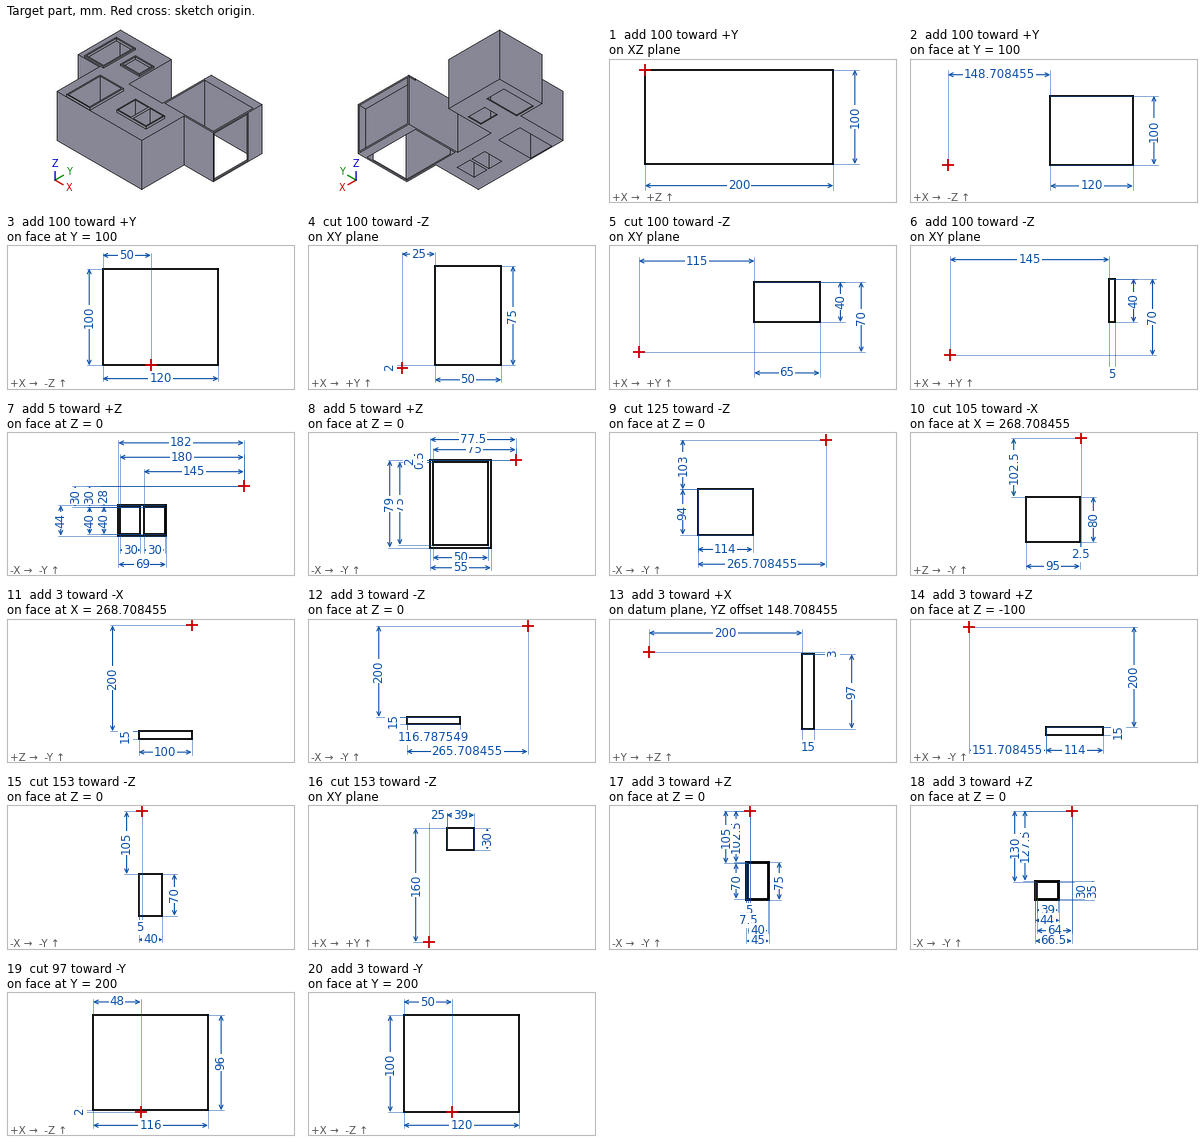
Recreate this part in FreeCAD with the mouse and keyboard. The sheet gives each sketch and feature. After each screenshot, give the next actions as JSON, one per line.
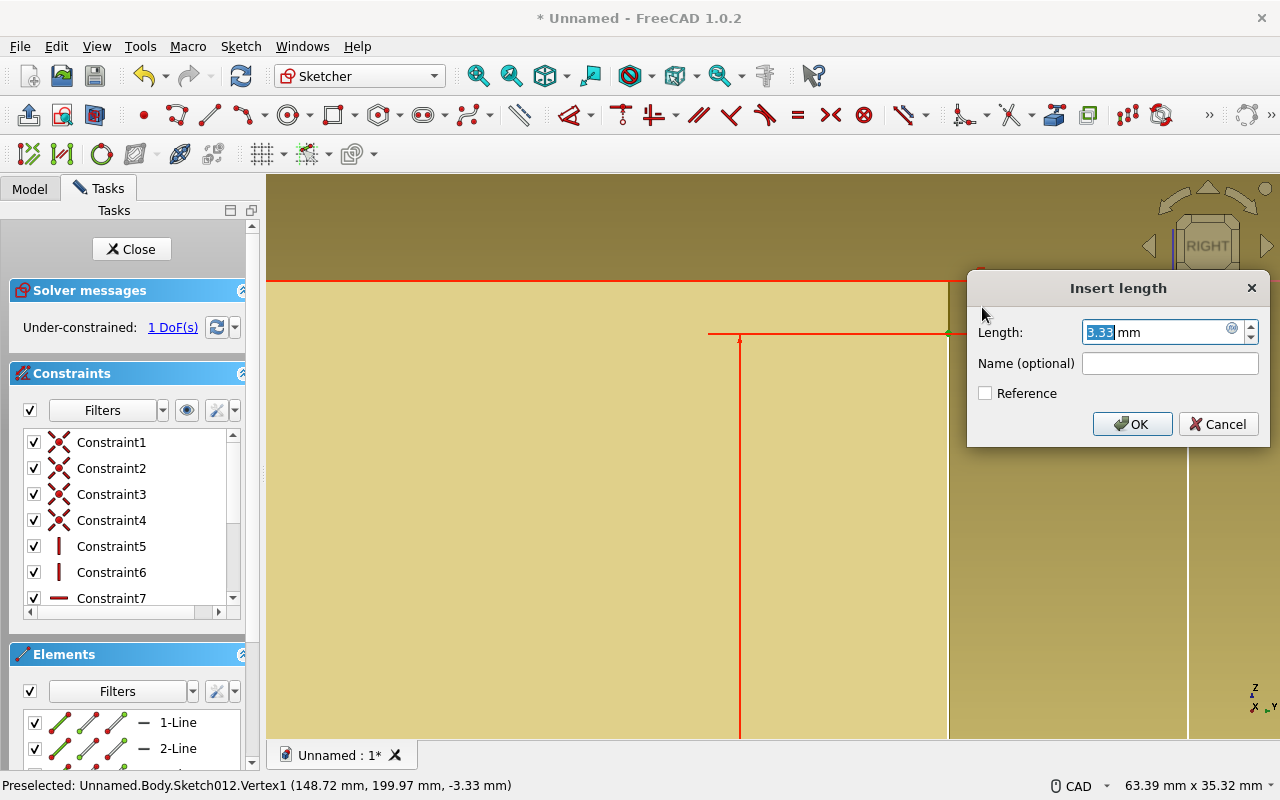
{"action": "type", "text": "3"}
{"action": "key", "text": "Return"}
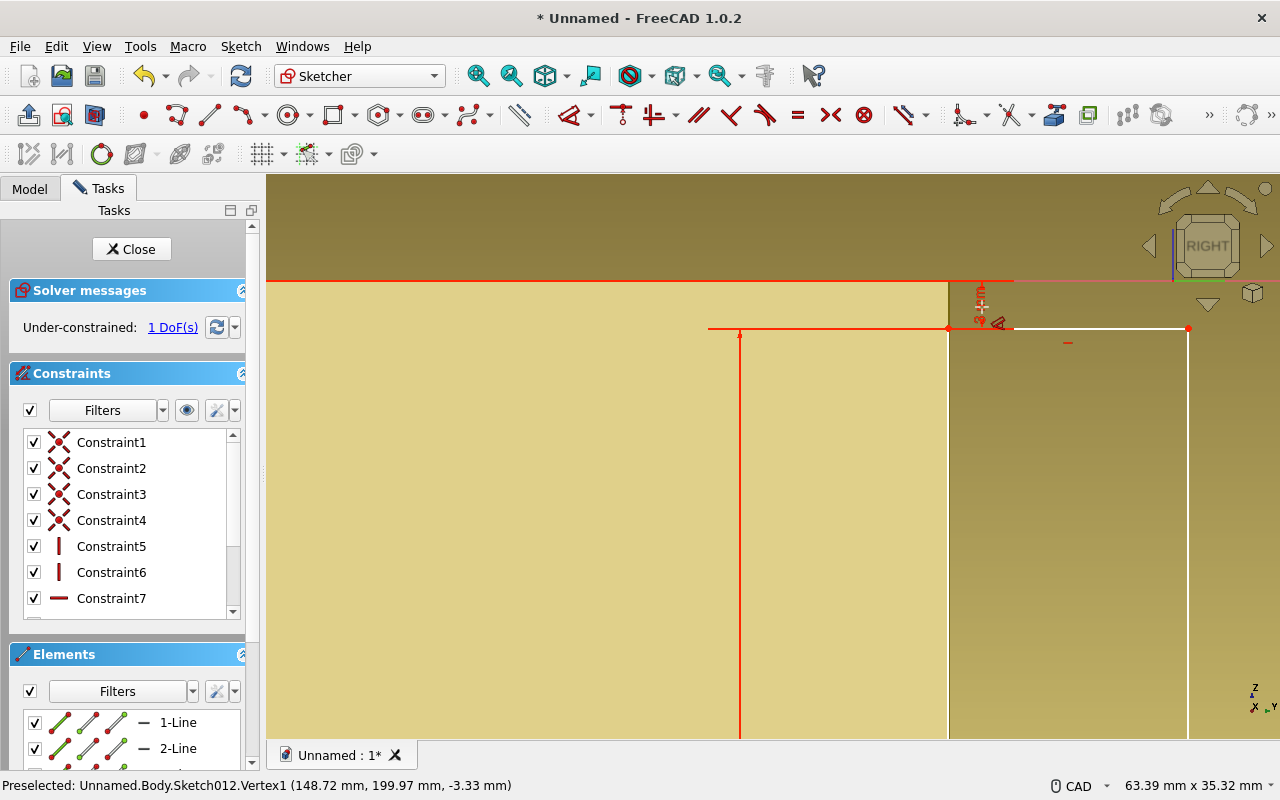
{"action": "scroll", "coordinate": [949, 333], "scroll_direction": "down", "scroll_amount": 9}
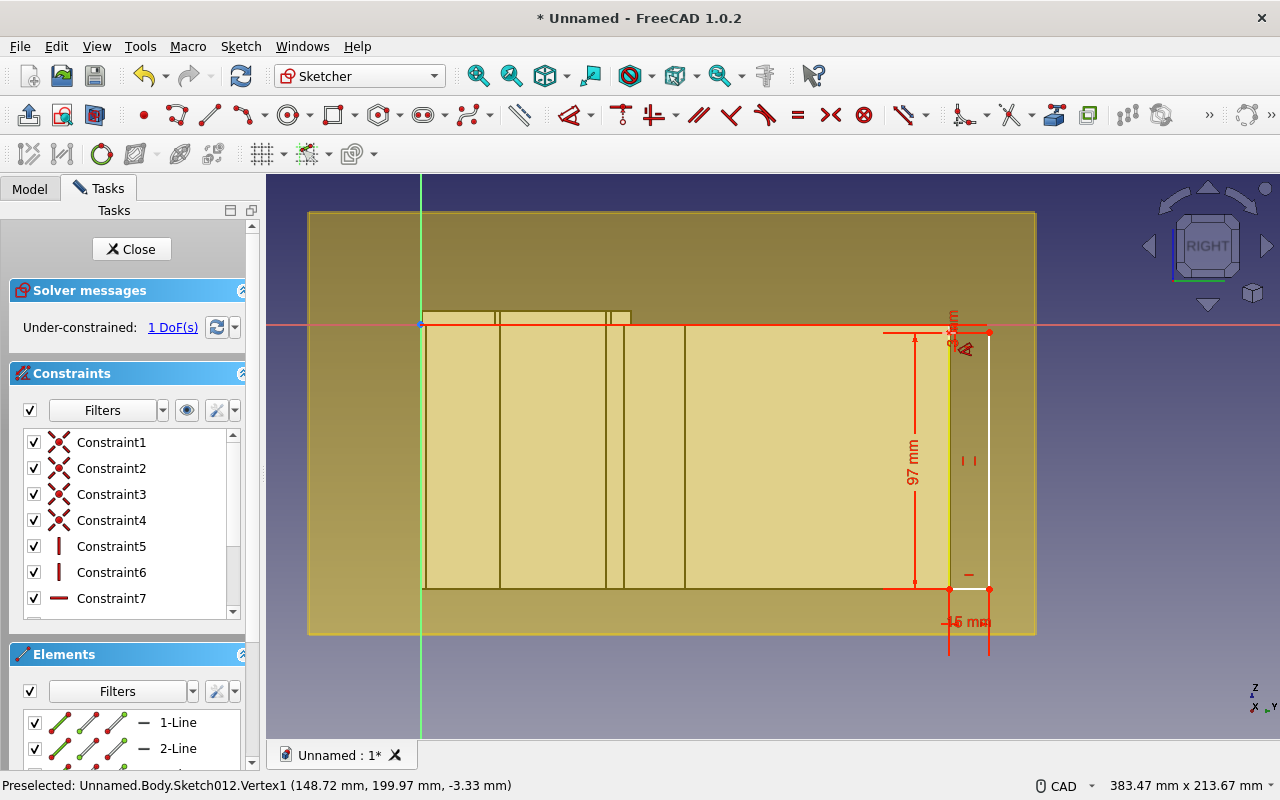
{"action": "left_click", "coordinate": [949, 333]}
{"action": "left_click", "coordinate": [685, 291]}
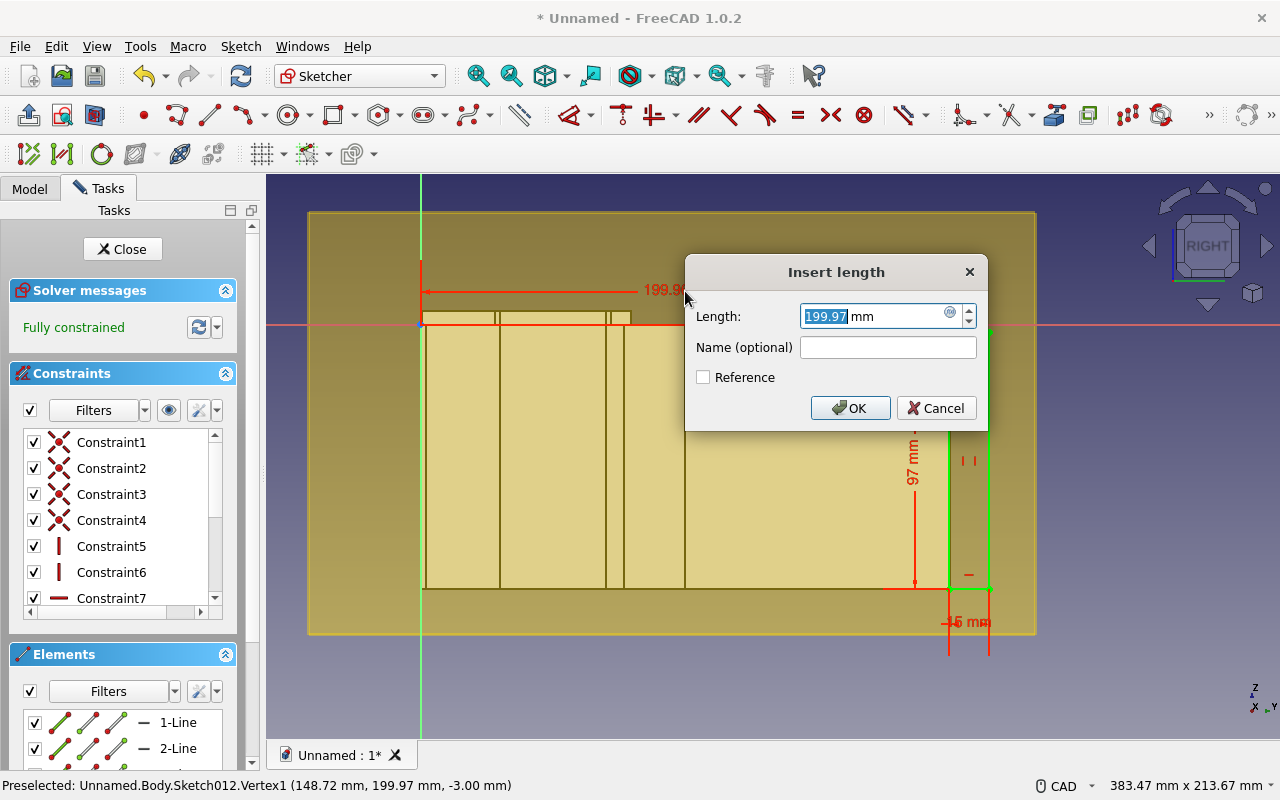
{"action": "type", "text": "200"}
{"action": "key", "text": "Return"}
{"action": "key", "text": "Escape"}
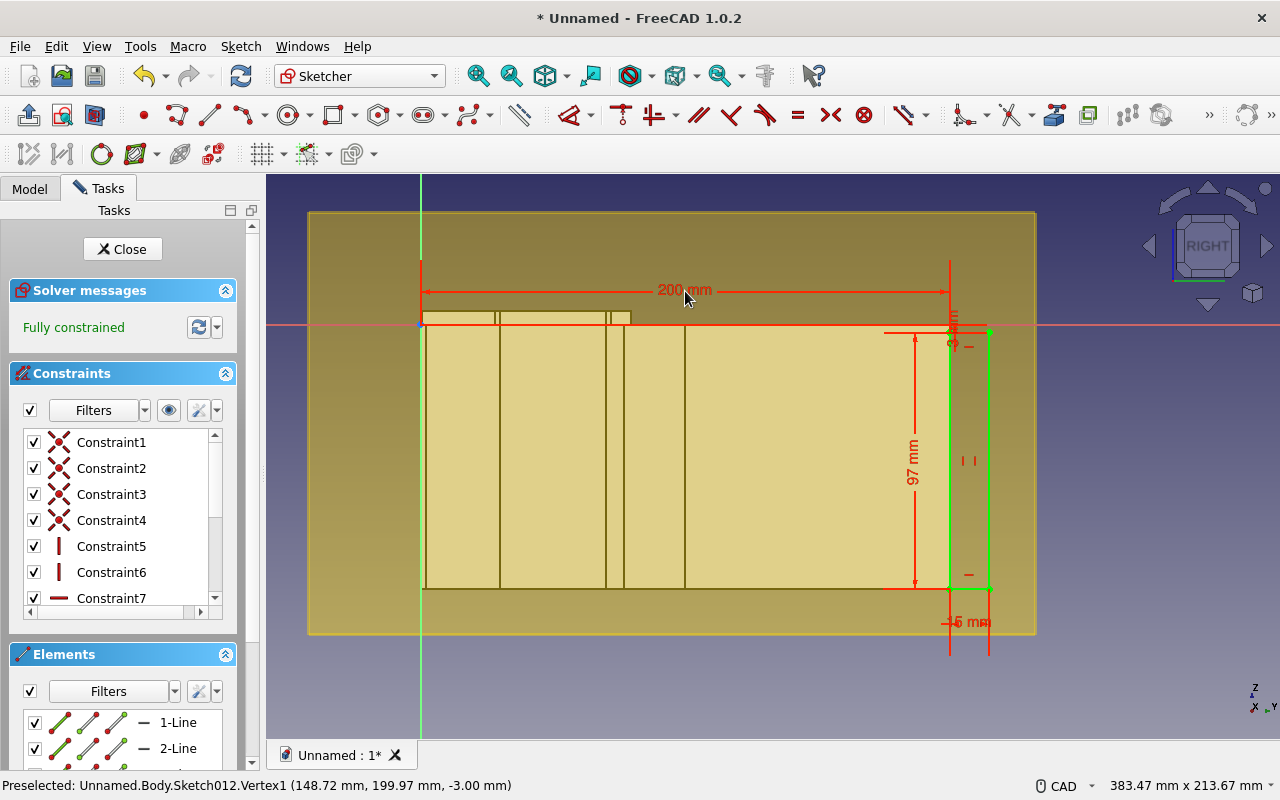
{"action": "left_click", "coordinate": [123, 249]}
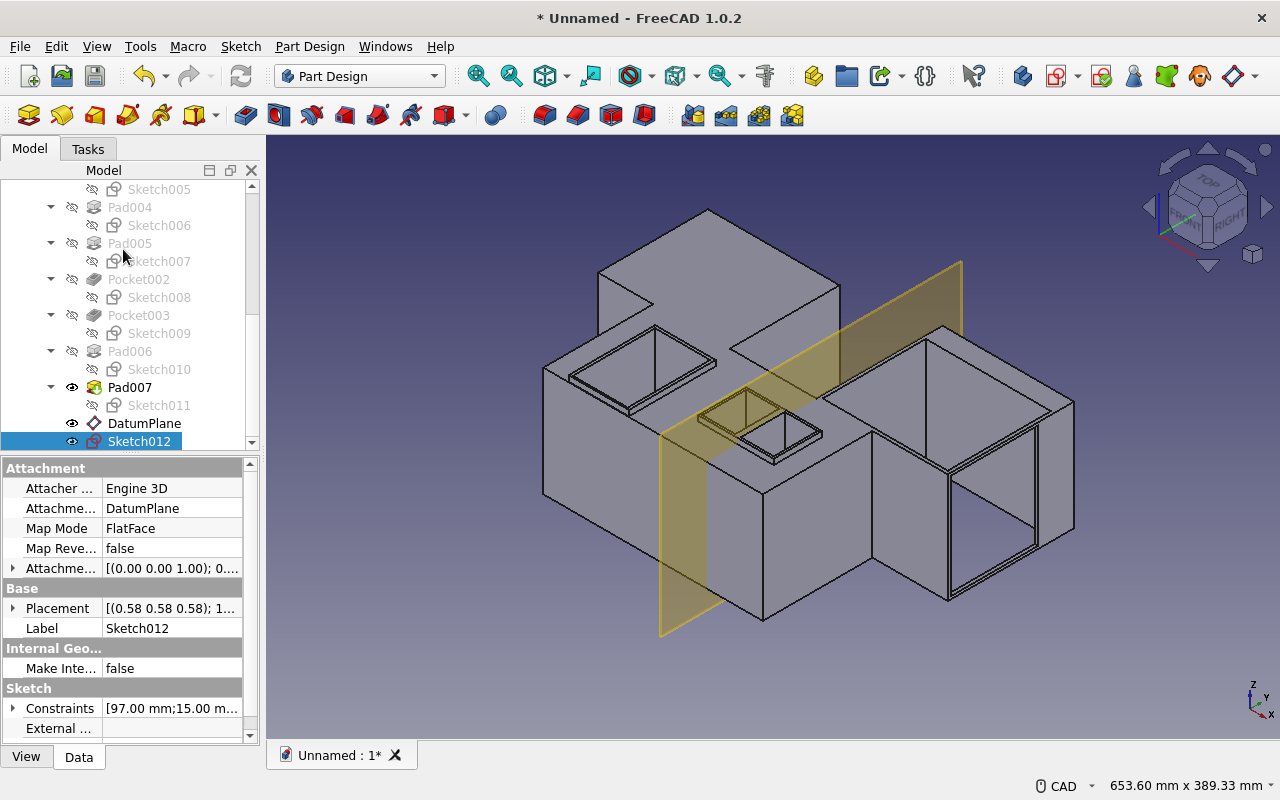
{"action": "left_click", "coordinate": [29, 116]}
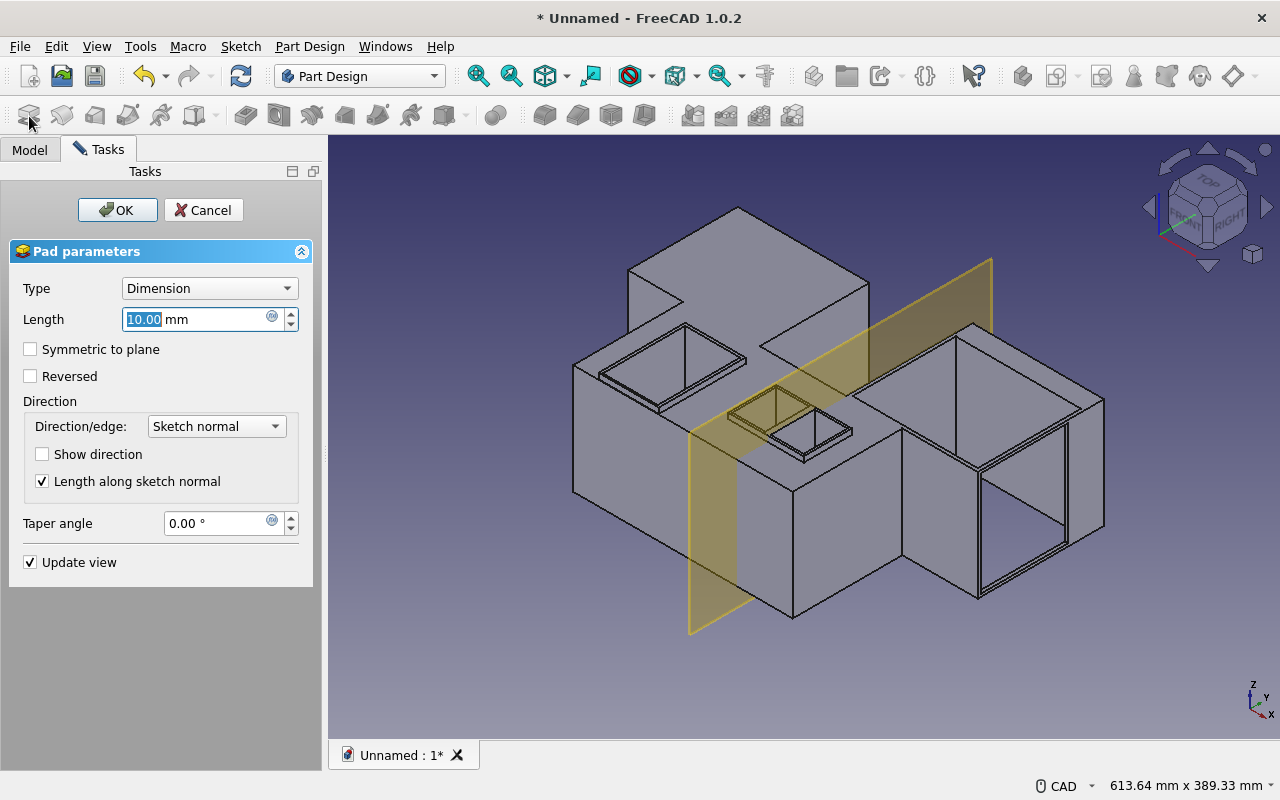
{"action": "type", "text": "3"}
{"action": "key", "text": "Tab"}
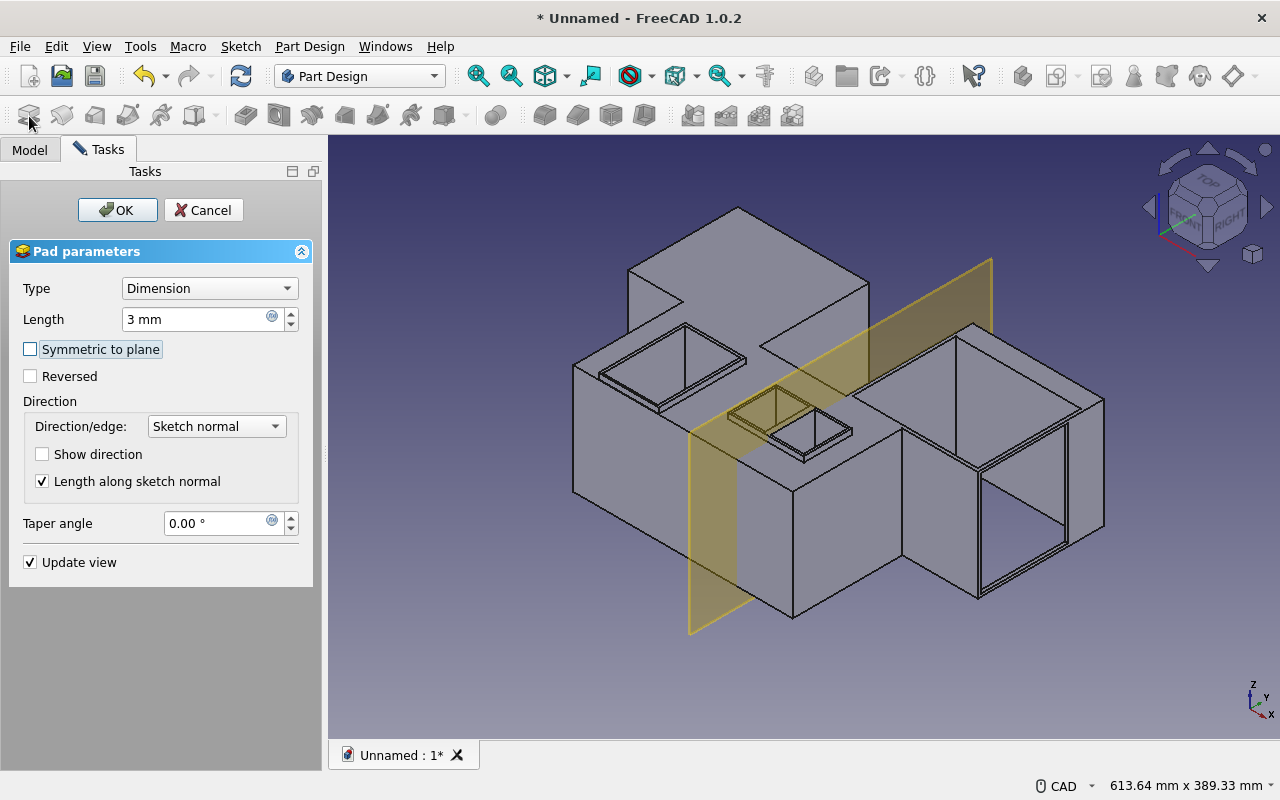
{"action": "left_click", "coordinate": [118, 210]}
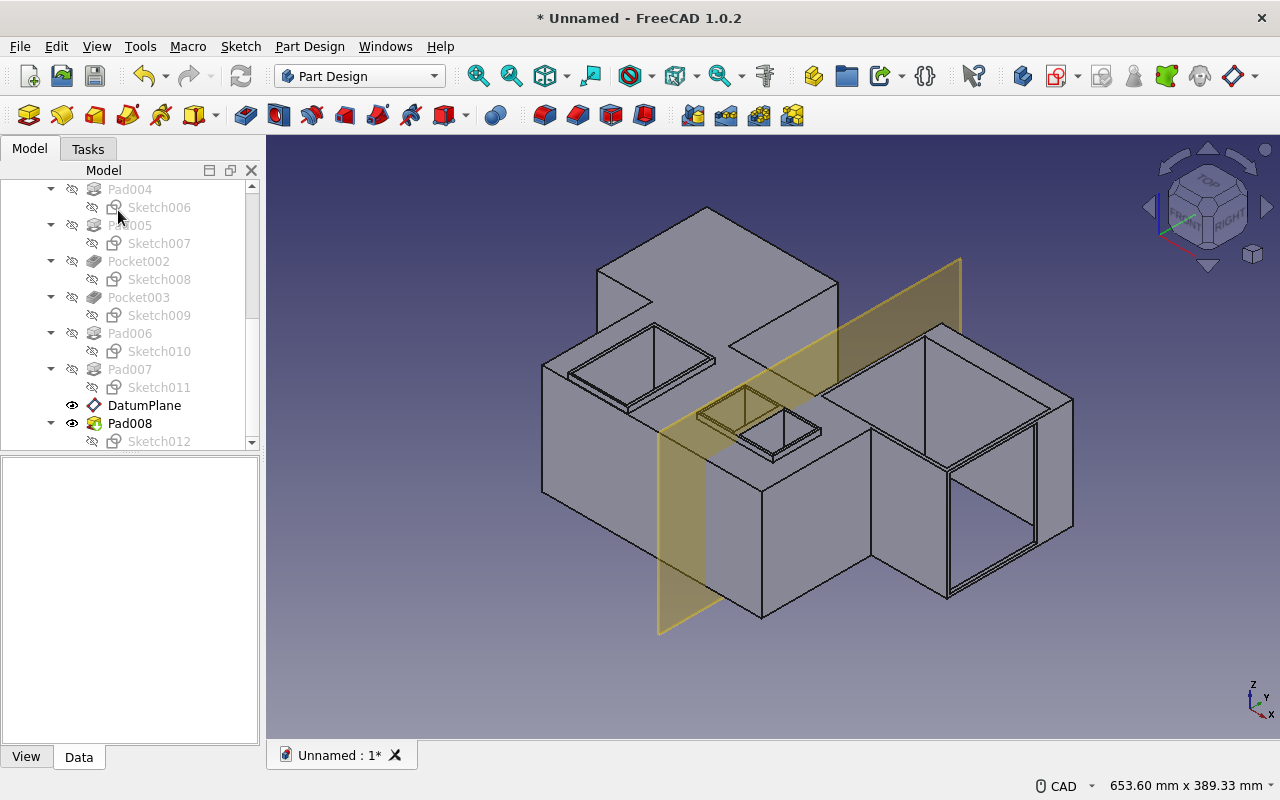
{"action": "left_click", "coordinate": [117, 405]}
{"action": "key", "text": "space"}